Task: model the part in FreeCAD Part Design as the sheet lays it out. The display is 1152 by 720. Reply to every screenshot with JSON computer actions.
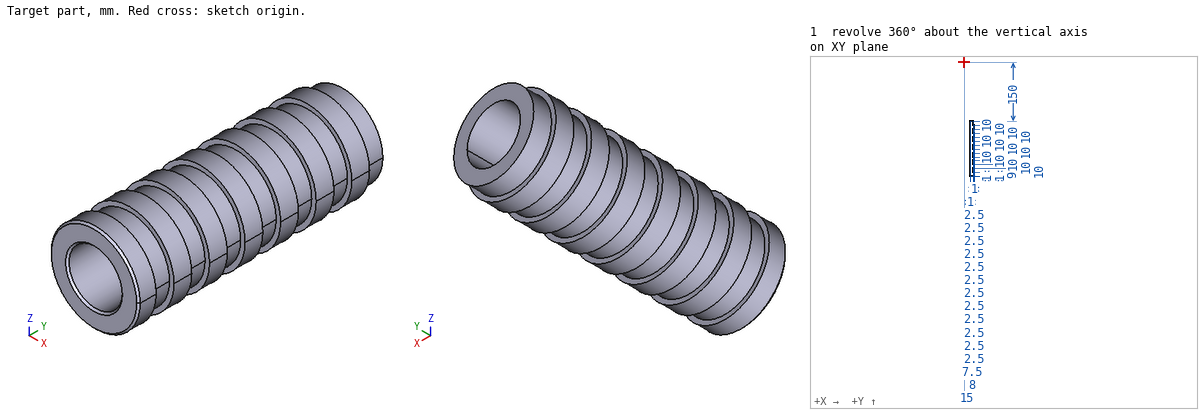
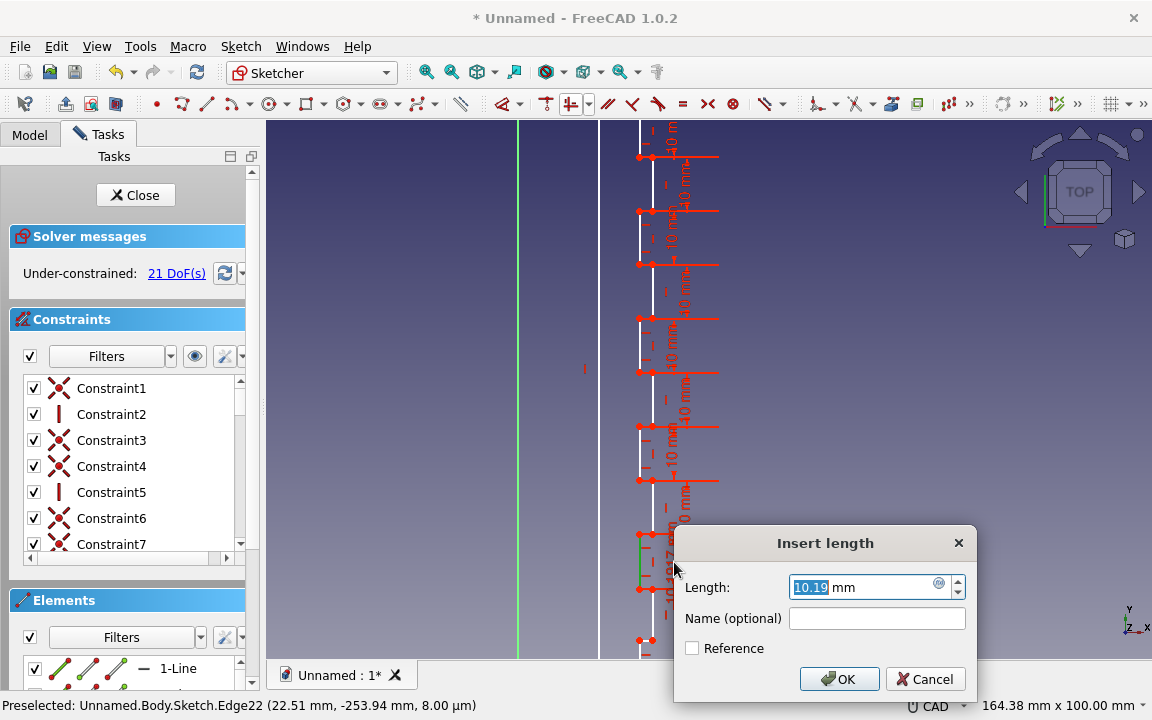
{"action": "type", "text": "10"}
{"action": "key", "text": "Return"}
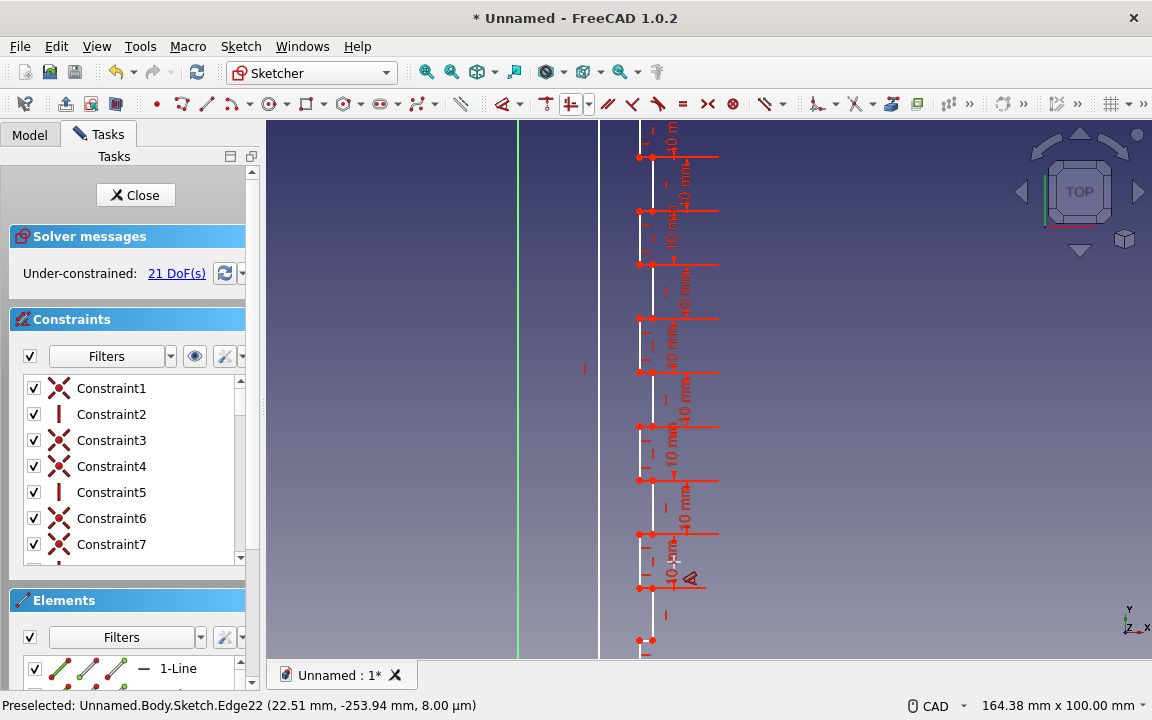
{"action": "left_click", "coordinate": [653, 604]}
{"action": "left_click", "coordinate": [687, 610]}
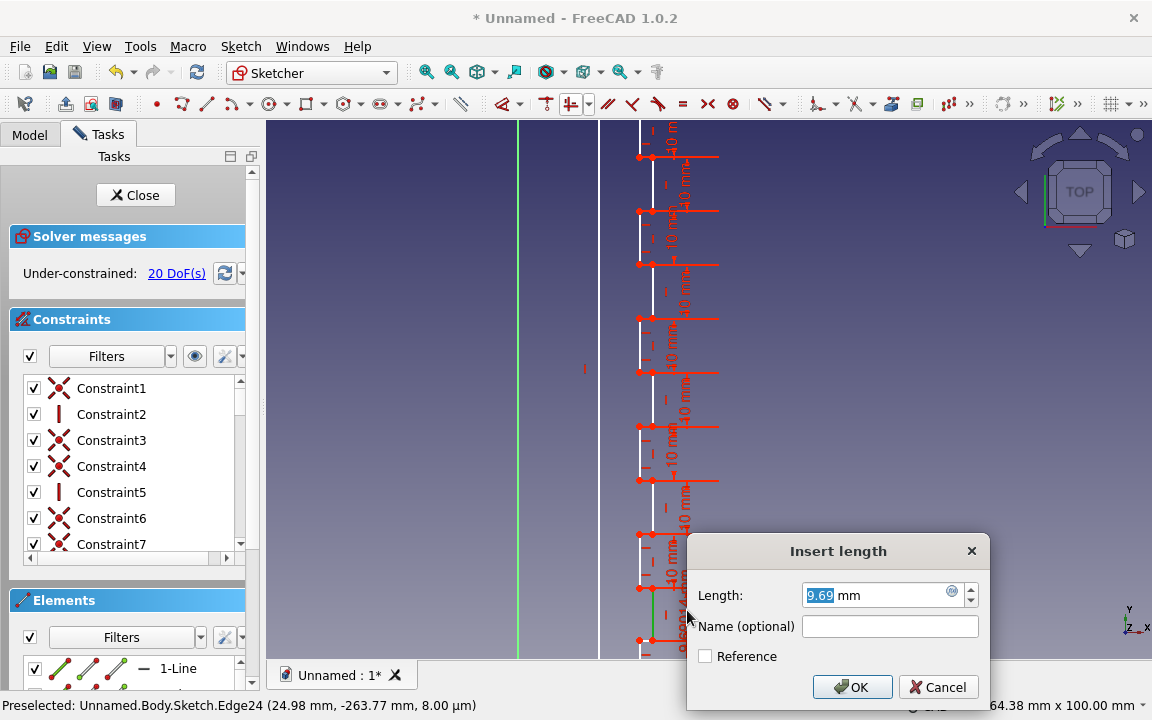
{"action": "type", "text": "10"}
{"action": "key", "text": "Return"}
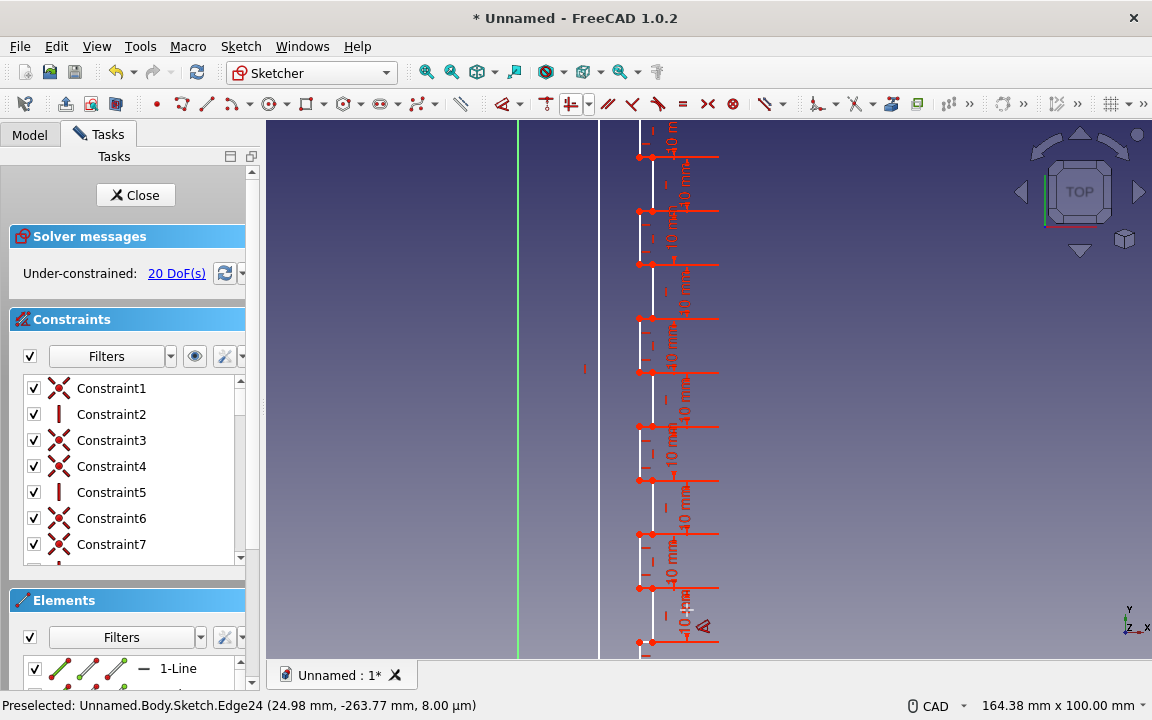
{"action": "scroll", "coordinate": [654, 497], "scroll_direction": "down", "scroll_amount": 8}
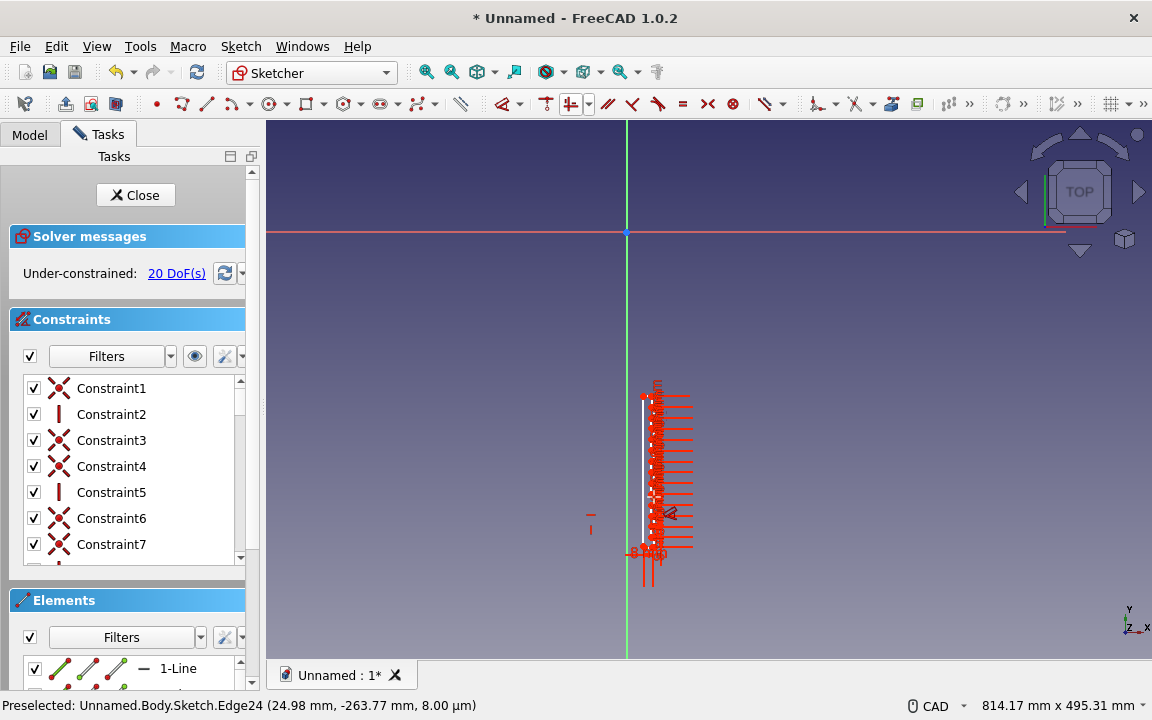
{"action": "scroll", "coordinate": [651, 530], "scroll_direction": "up", "scroll_amount": 8}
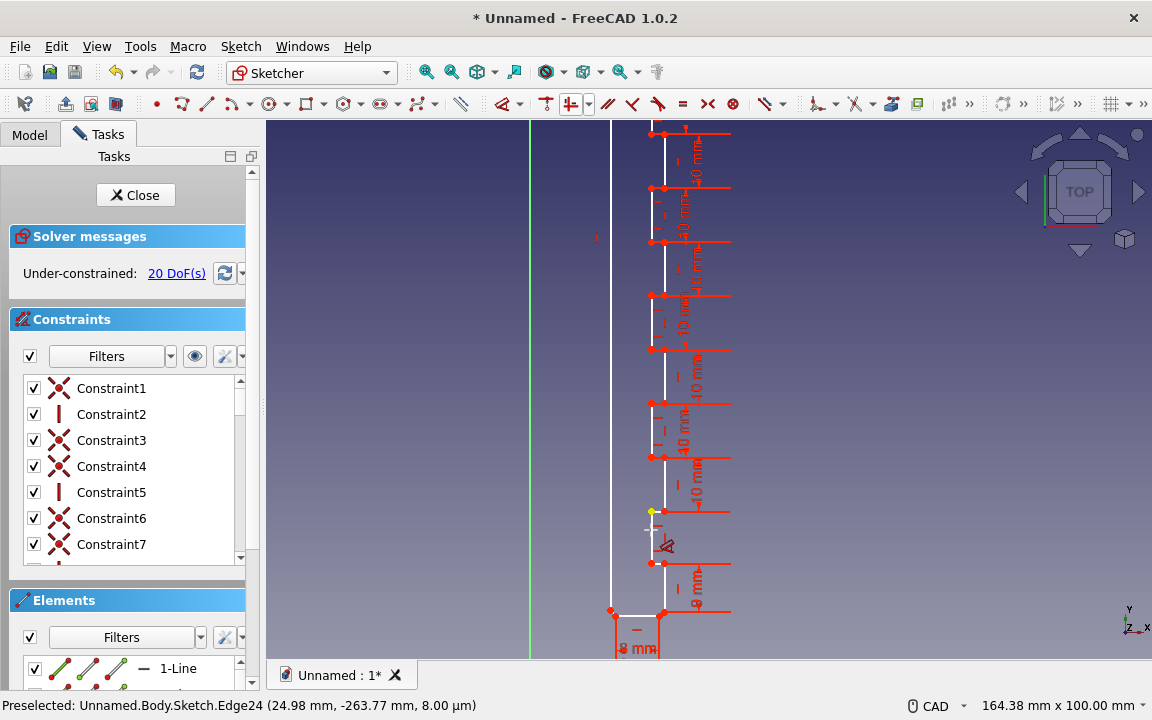
{"action": "left_click", "coordinate": [652, 527]}
{"action": "left_click", "coordinate": [686, 538]}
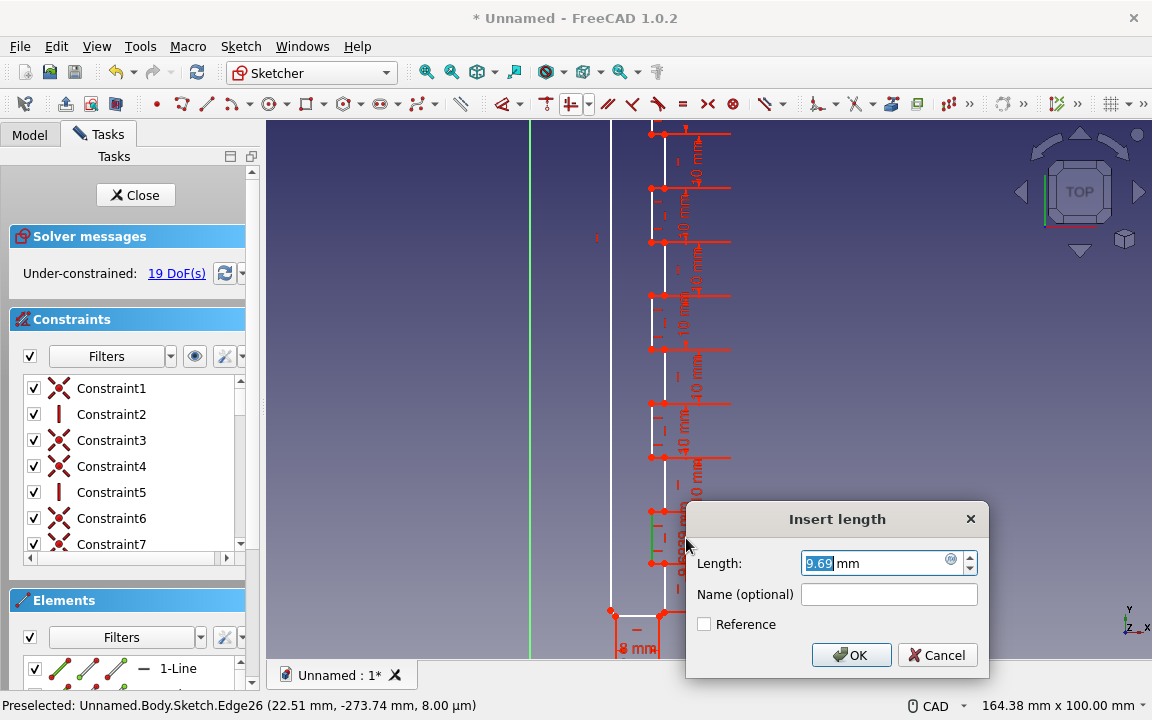
{"action": "type", "text": "10"}
{"action": "key", "text": "Return"}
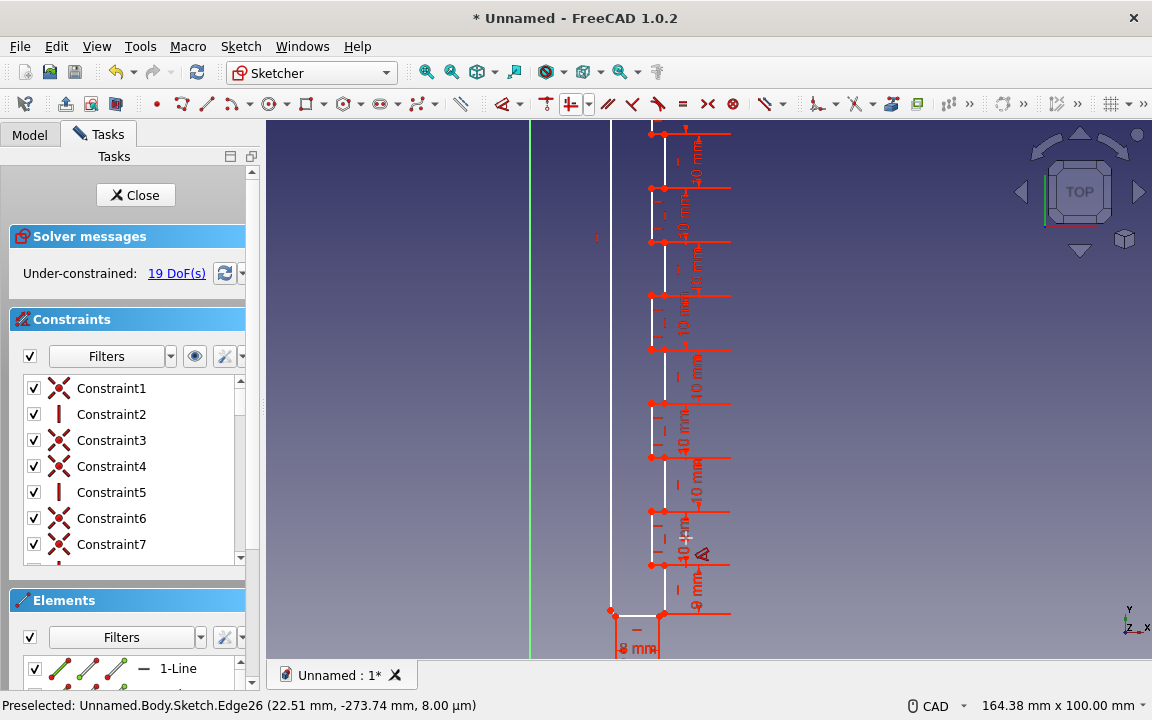
{"action": "scroll", "coordinate": [662, 615], "scroll_direction": "up", "scroll_amount": 10}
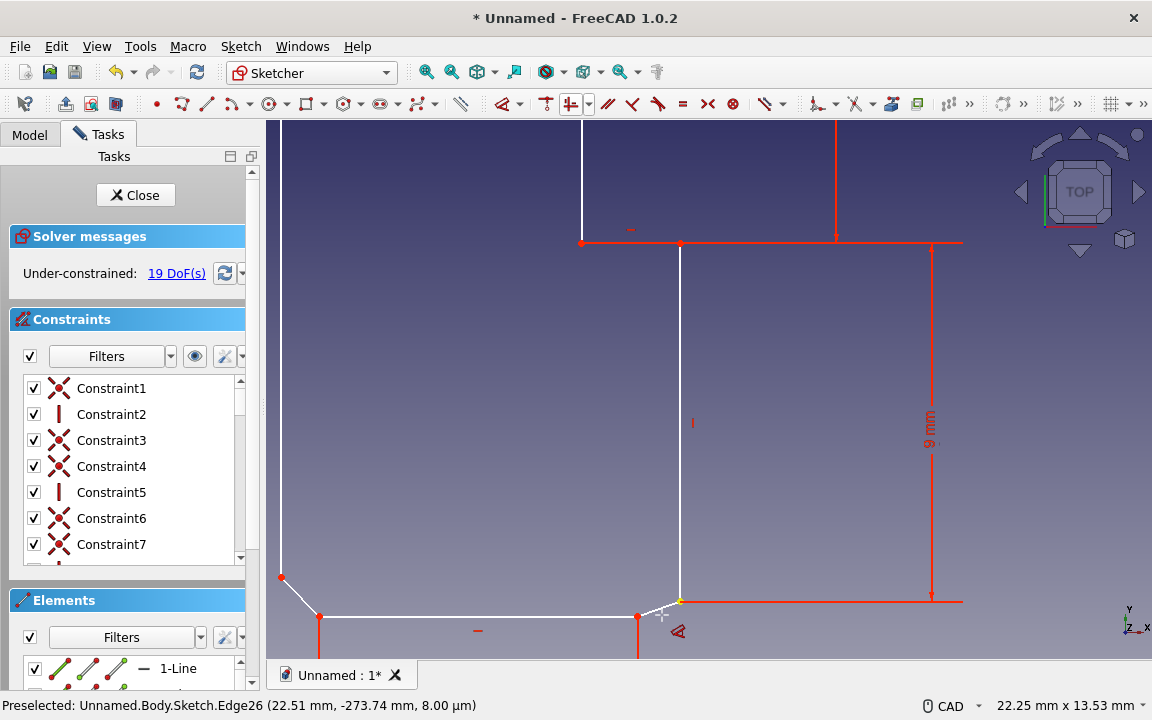
{"action": "left_click", "coordinate": [659, 609]}
{"action": "left_click", "coordinate": [659, 568]}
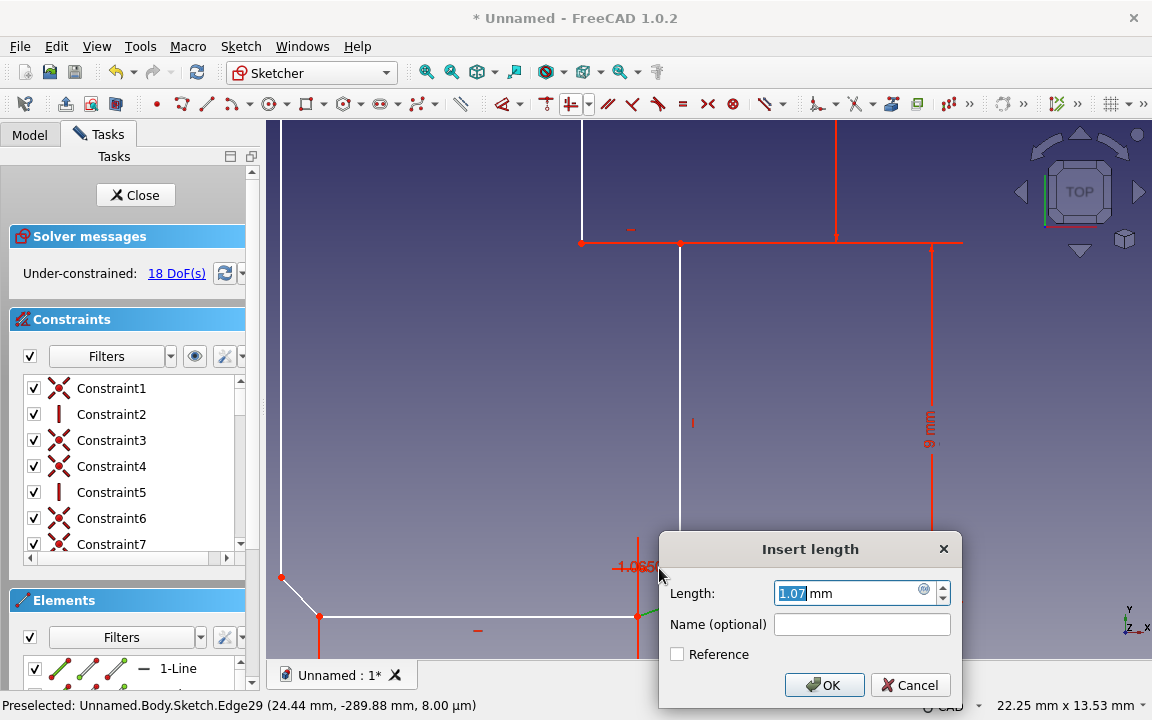
{"action": "type", "text": "1"}
{"action": "key", "text": "Return"}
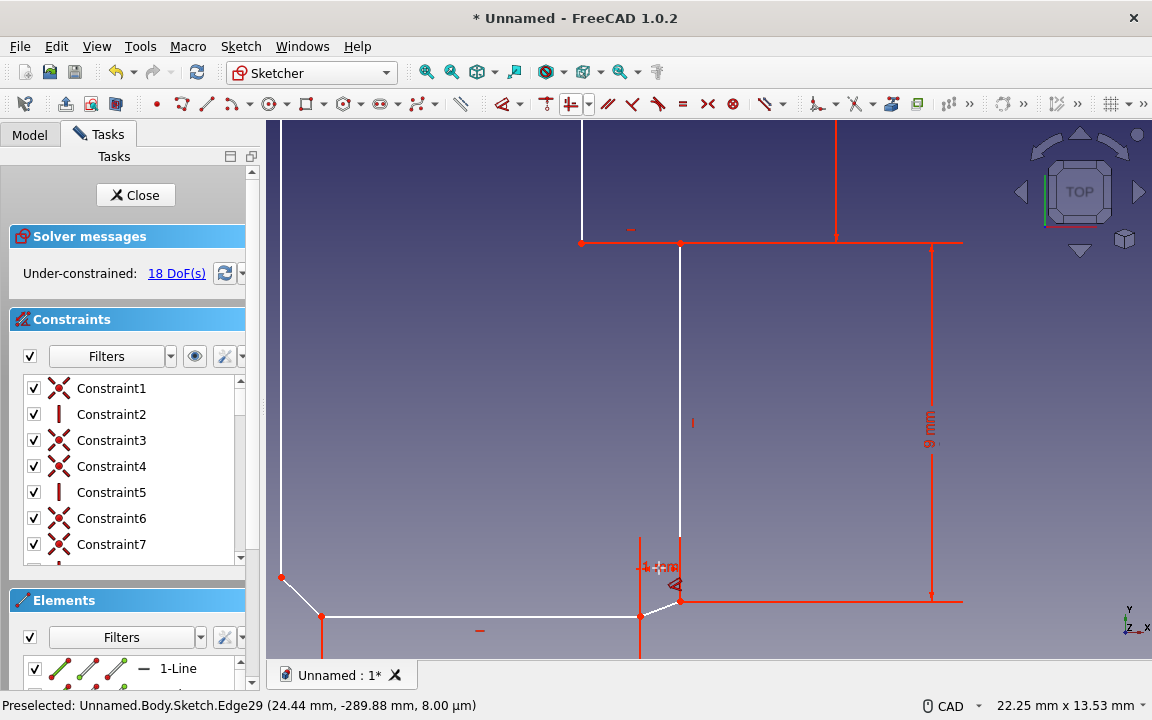
{"action": "left_click", "coordinate": [668, 606]}
{"action": "left_click", "coordinate": [714, 609]}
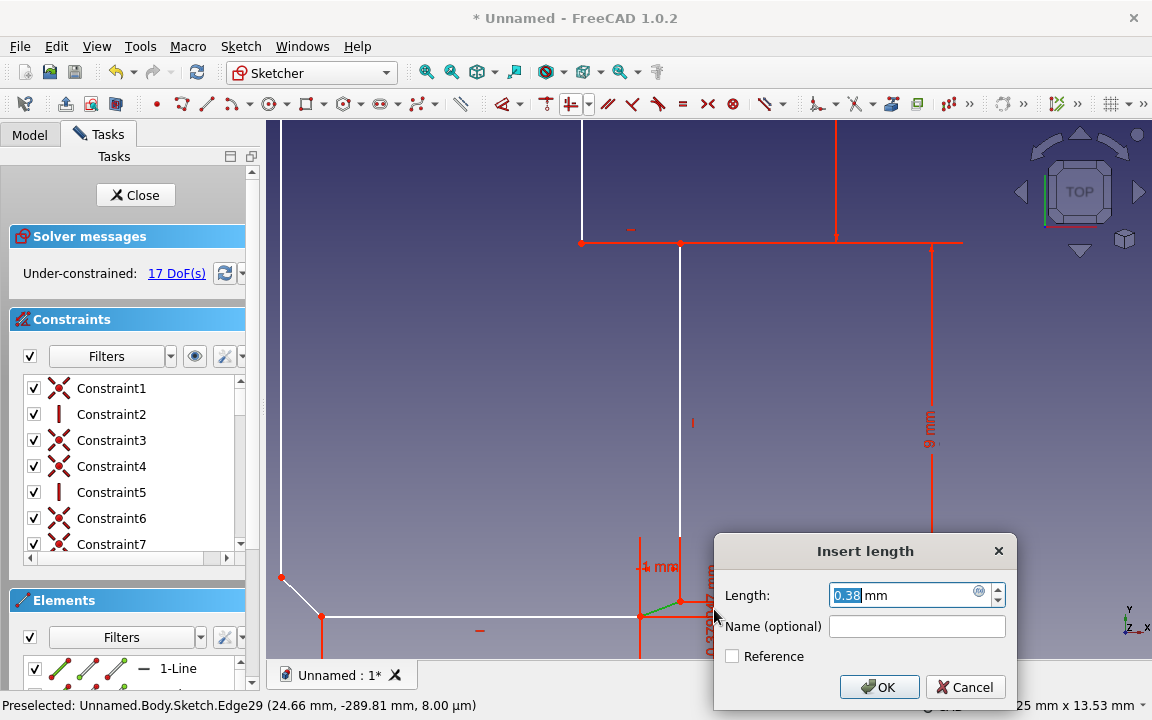
{"action": "type", "text": "1"}
{"action": "key", "text": "Return"}